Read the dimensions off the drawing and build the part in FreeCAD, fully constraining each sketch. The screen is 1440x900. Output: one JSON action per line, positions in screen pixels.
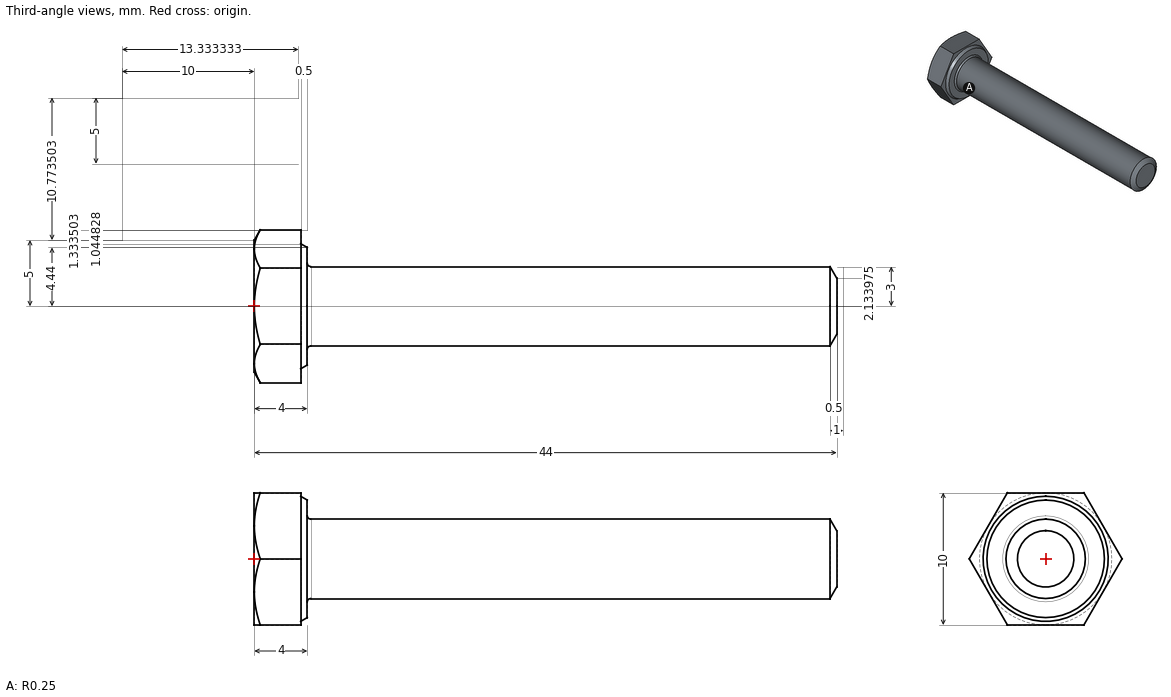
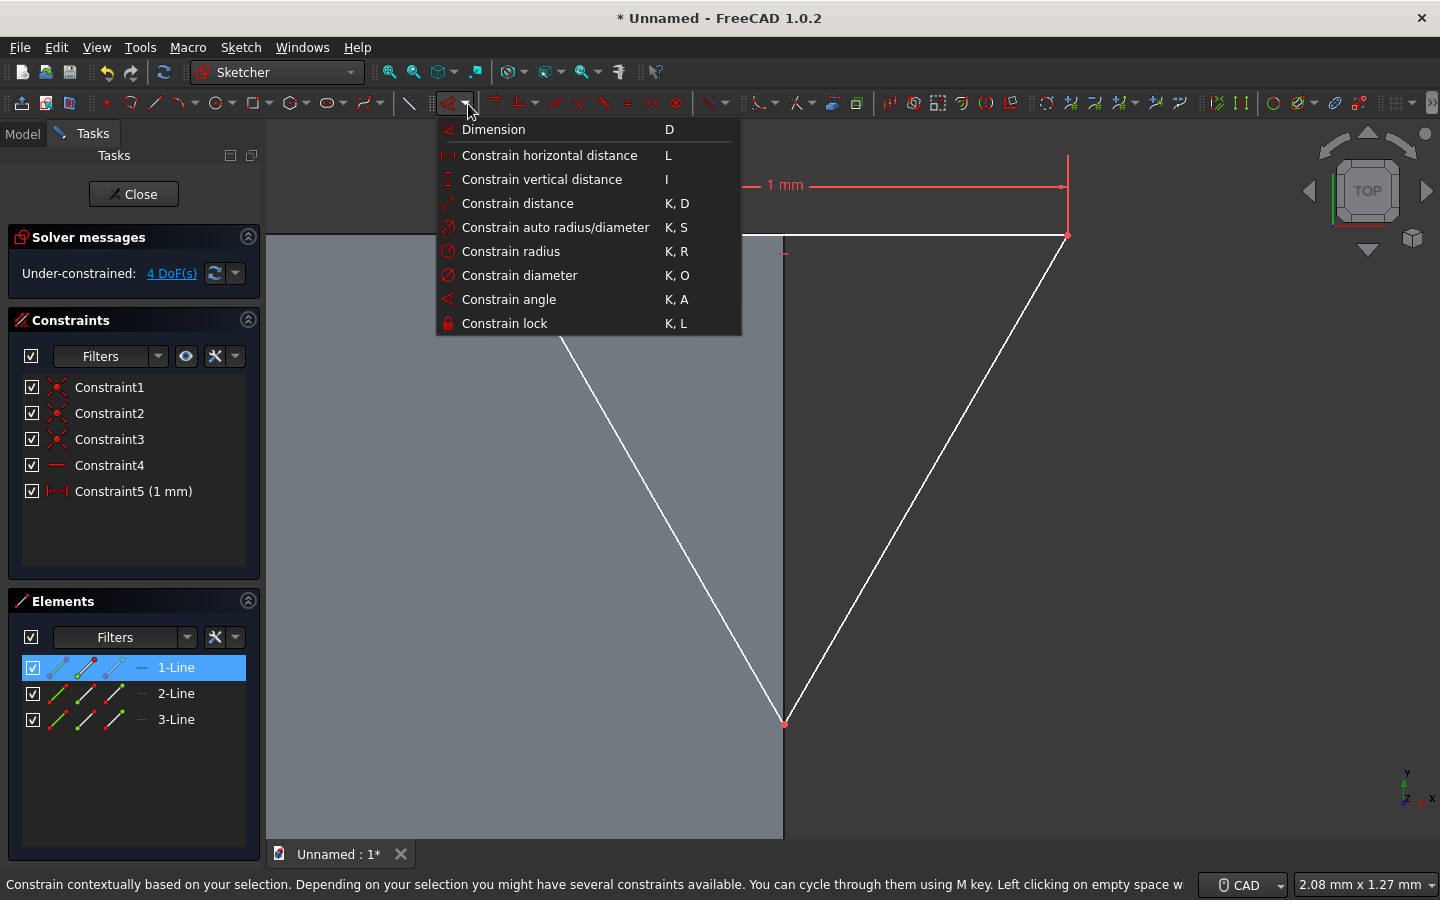
{"action": "left_click", "coordinate": [589, 179]}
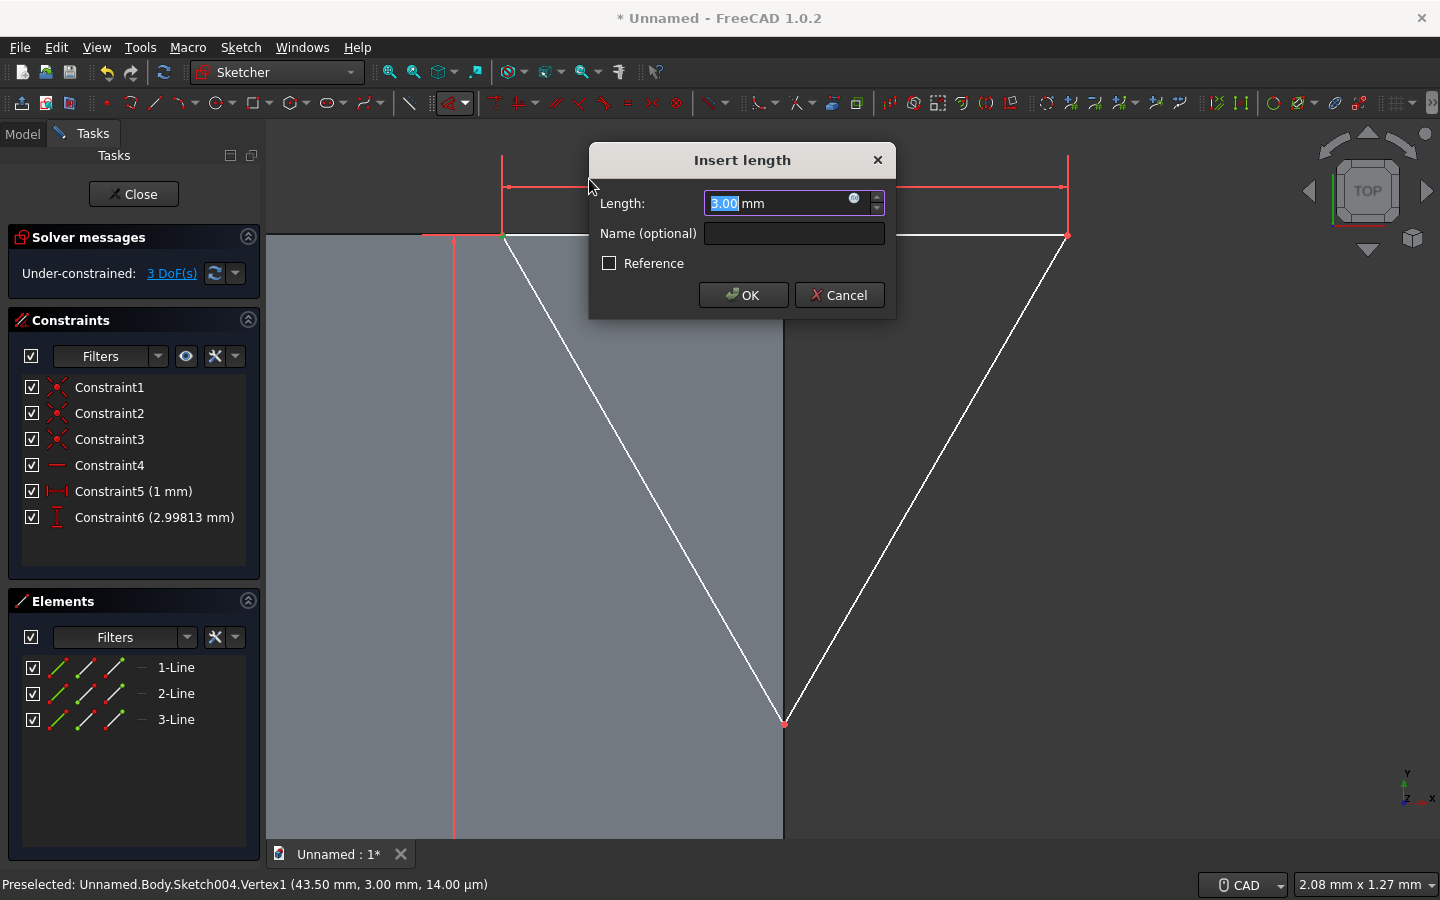
{"action": "type", "text": "3"}
{"action": "key", "text": "Return"}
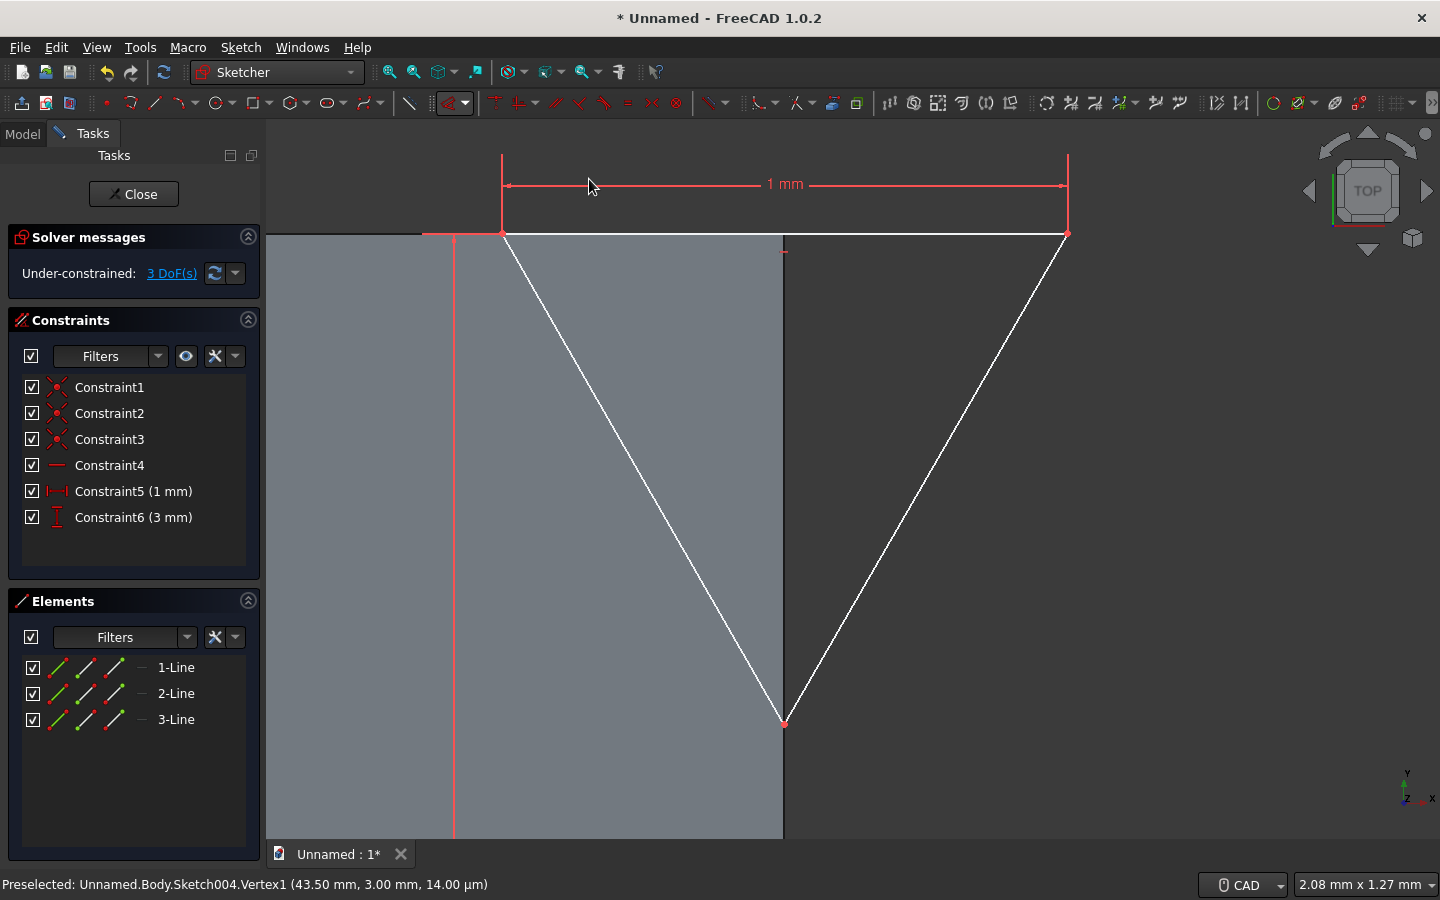
{"action": "left_click", "coordinate": [784, 725]}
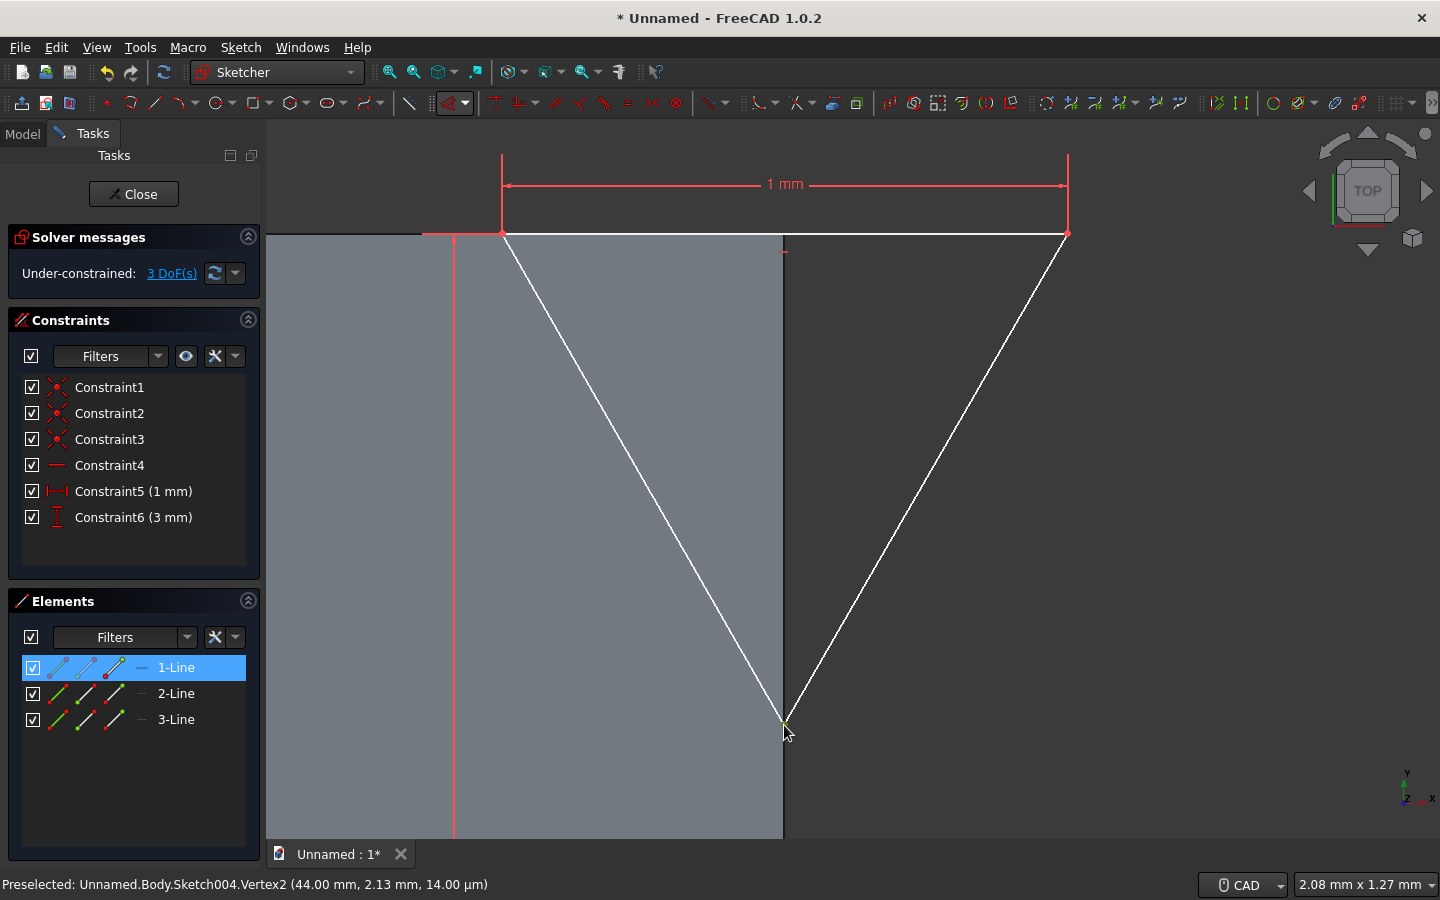
{"action": "left_click", "coordinate": [468, 104]}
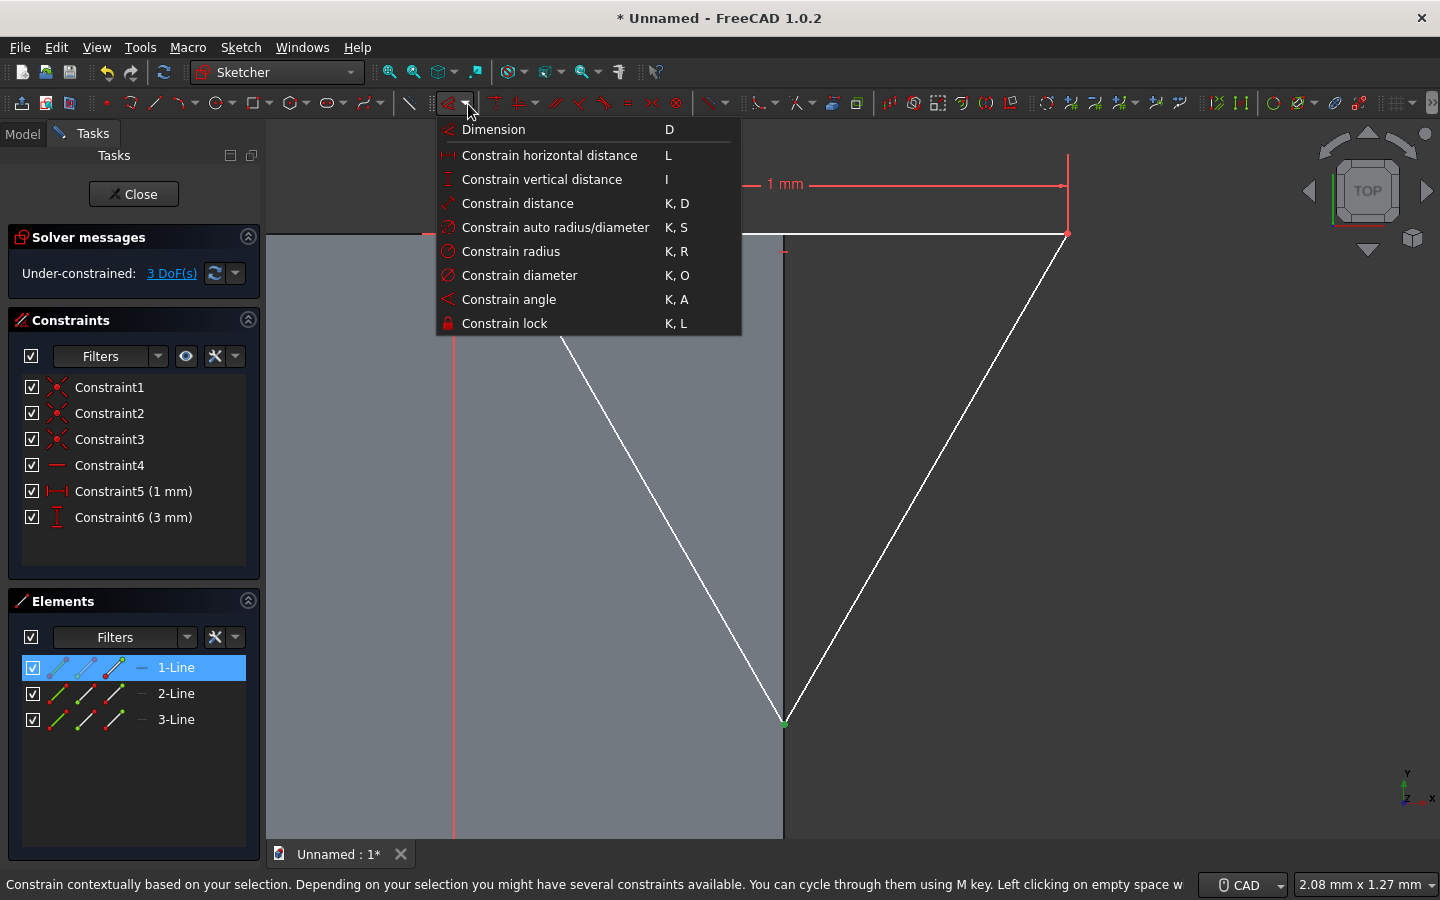
{"action": "left_click", "coordinate": [589, 155]}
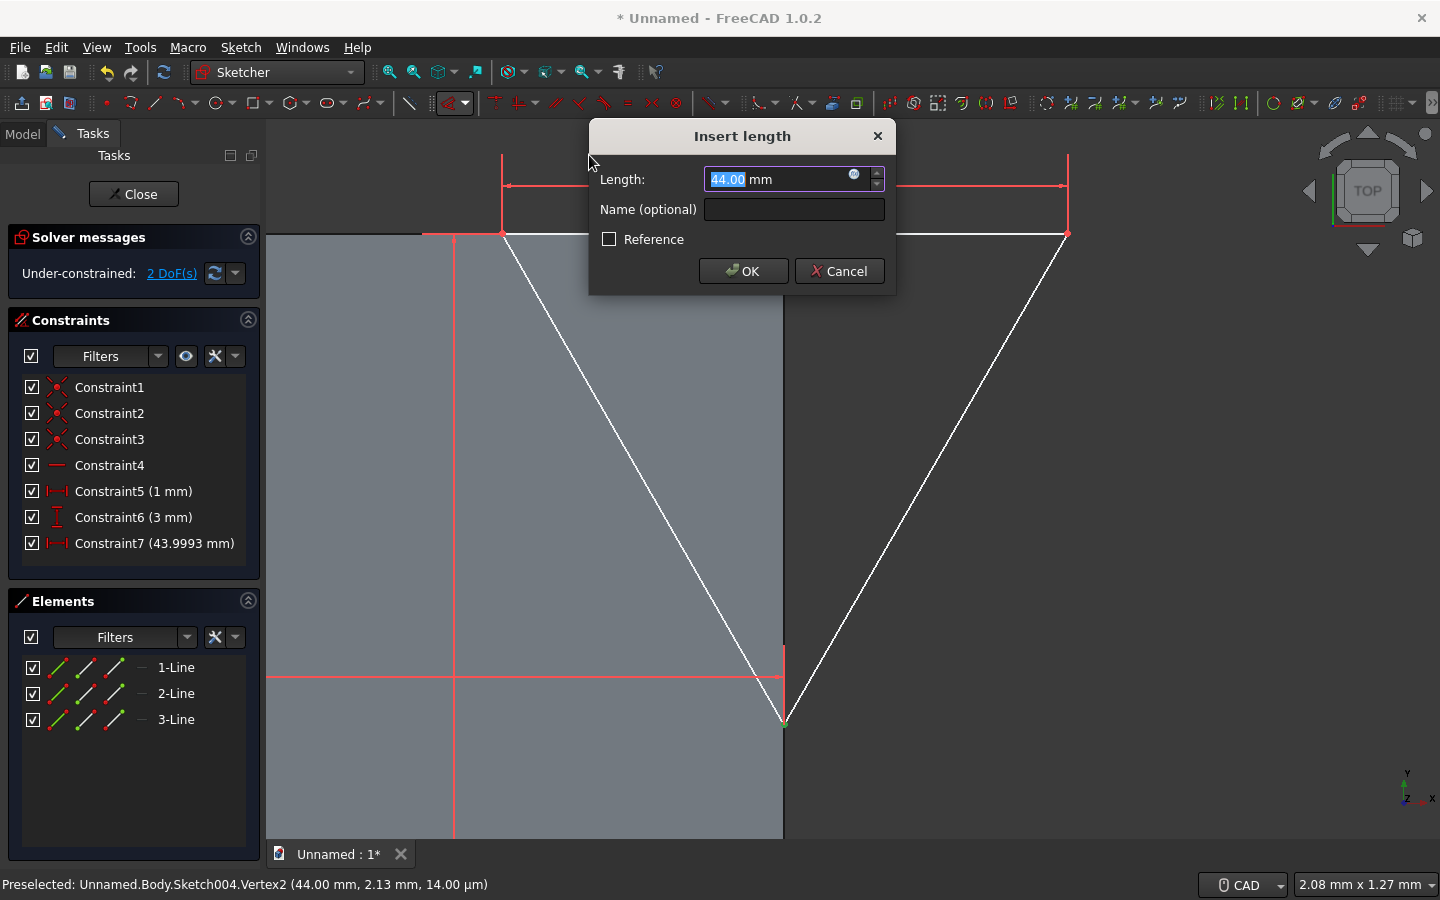
{"action": "type", "text": "44"}
{"action": "key", "text": "Return"}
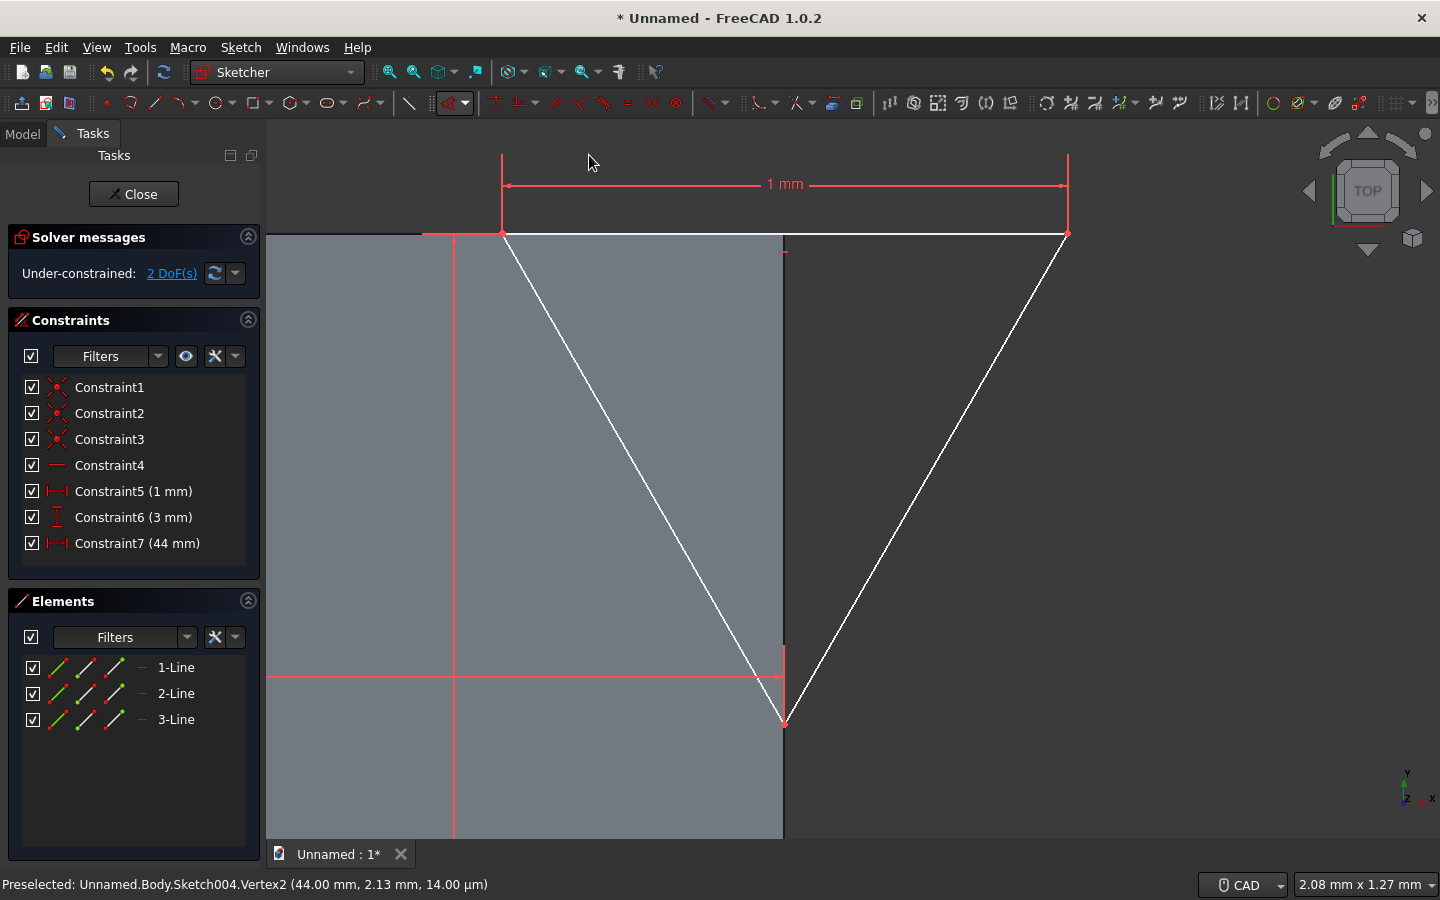
{"action": "left_click", "coordinate": [587, 381]}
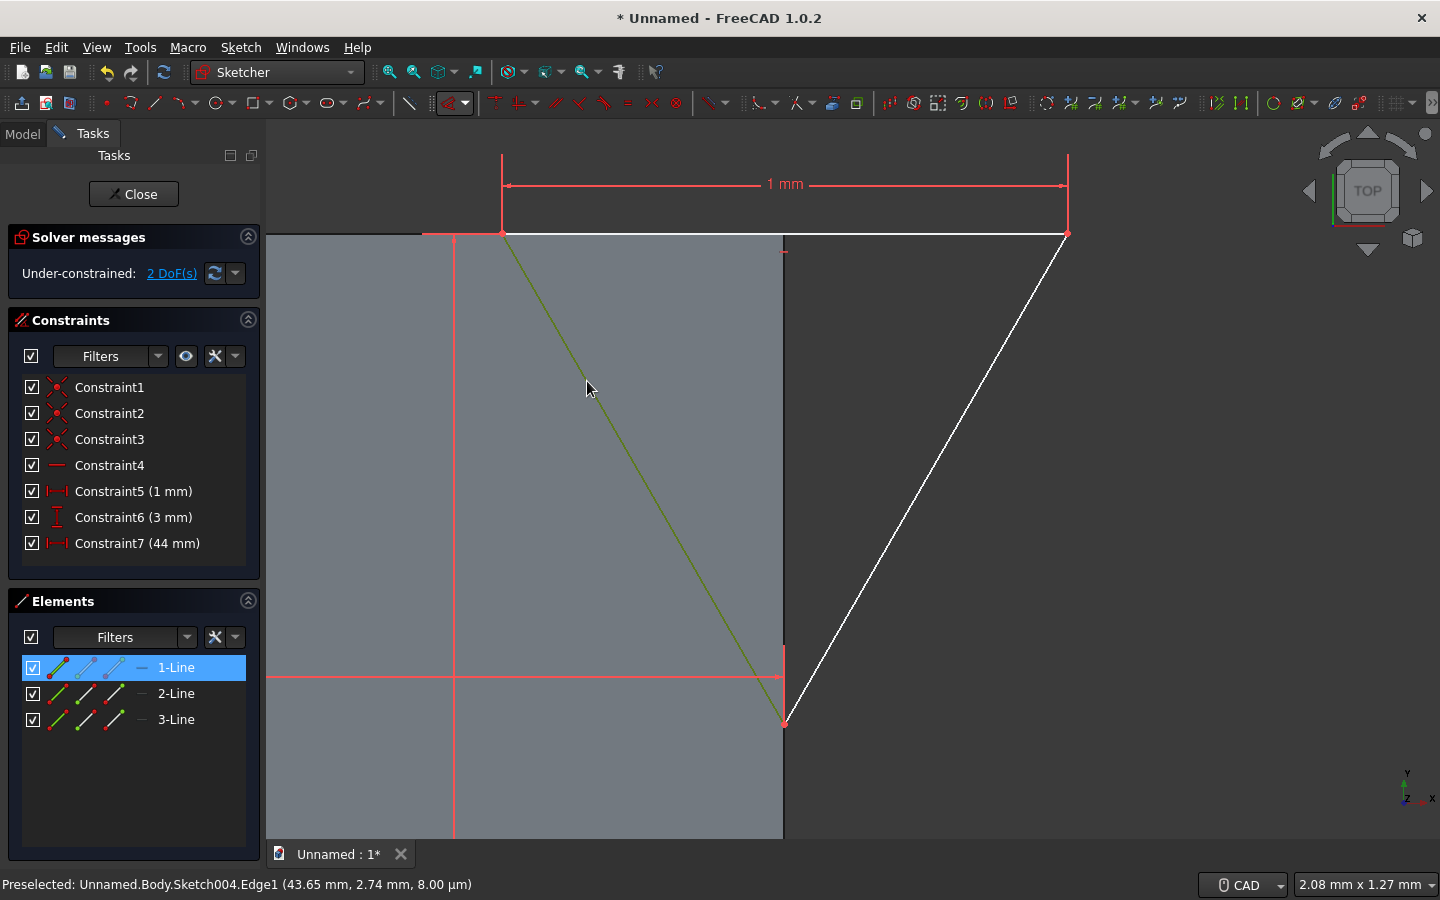
{"action": "left_click", "coordinate": [468, 104]}